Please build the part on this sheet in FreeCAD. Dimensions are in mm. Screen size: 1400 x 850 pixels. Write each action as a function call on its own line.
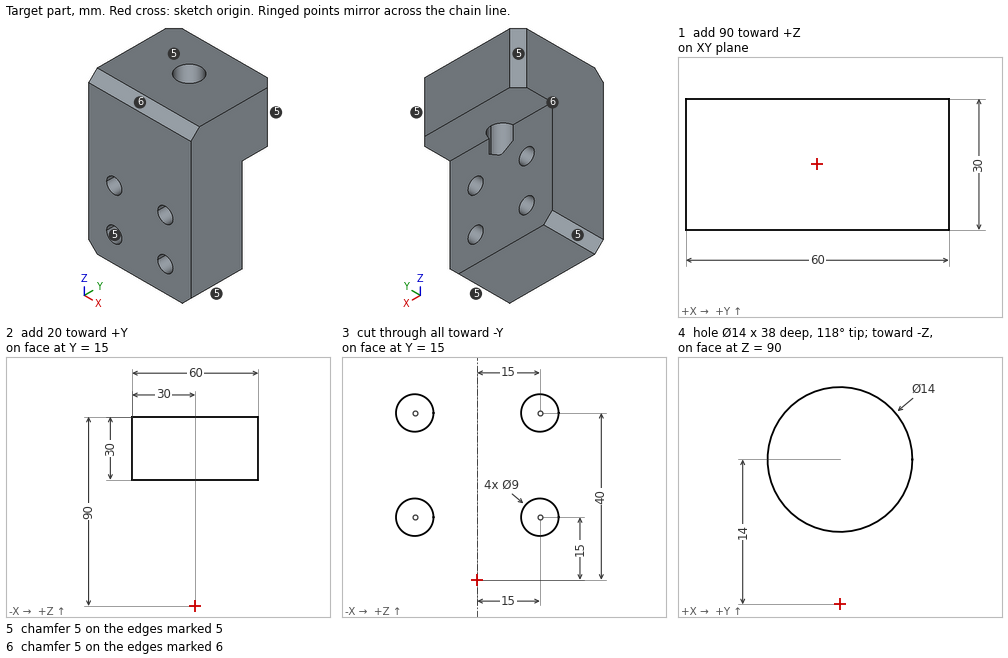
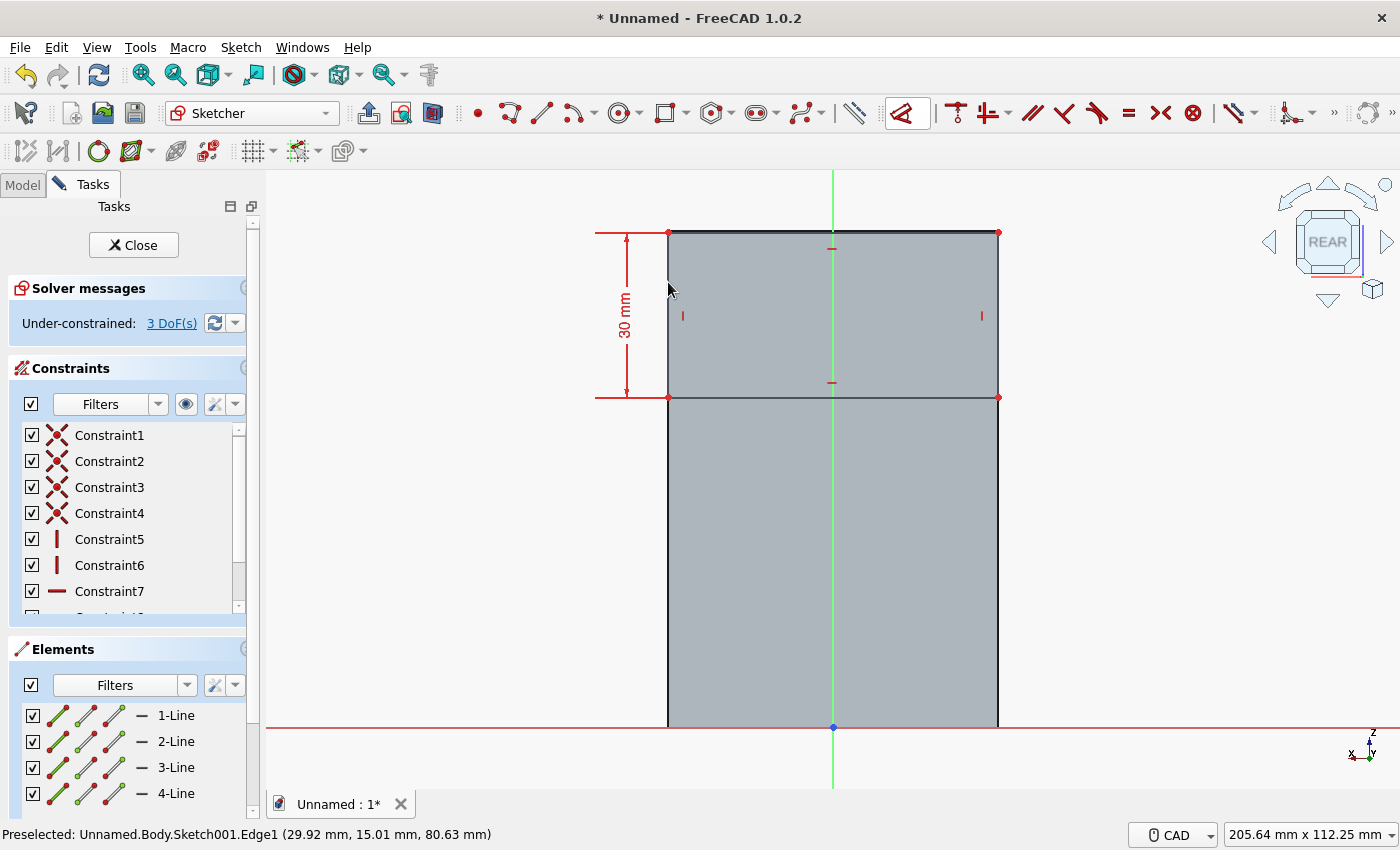
click(767, 398)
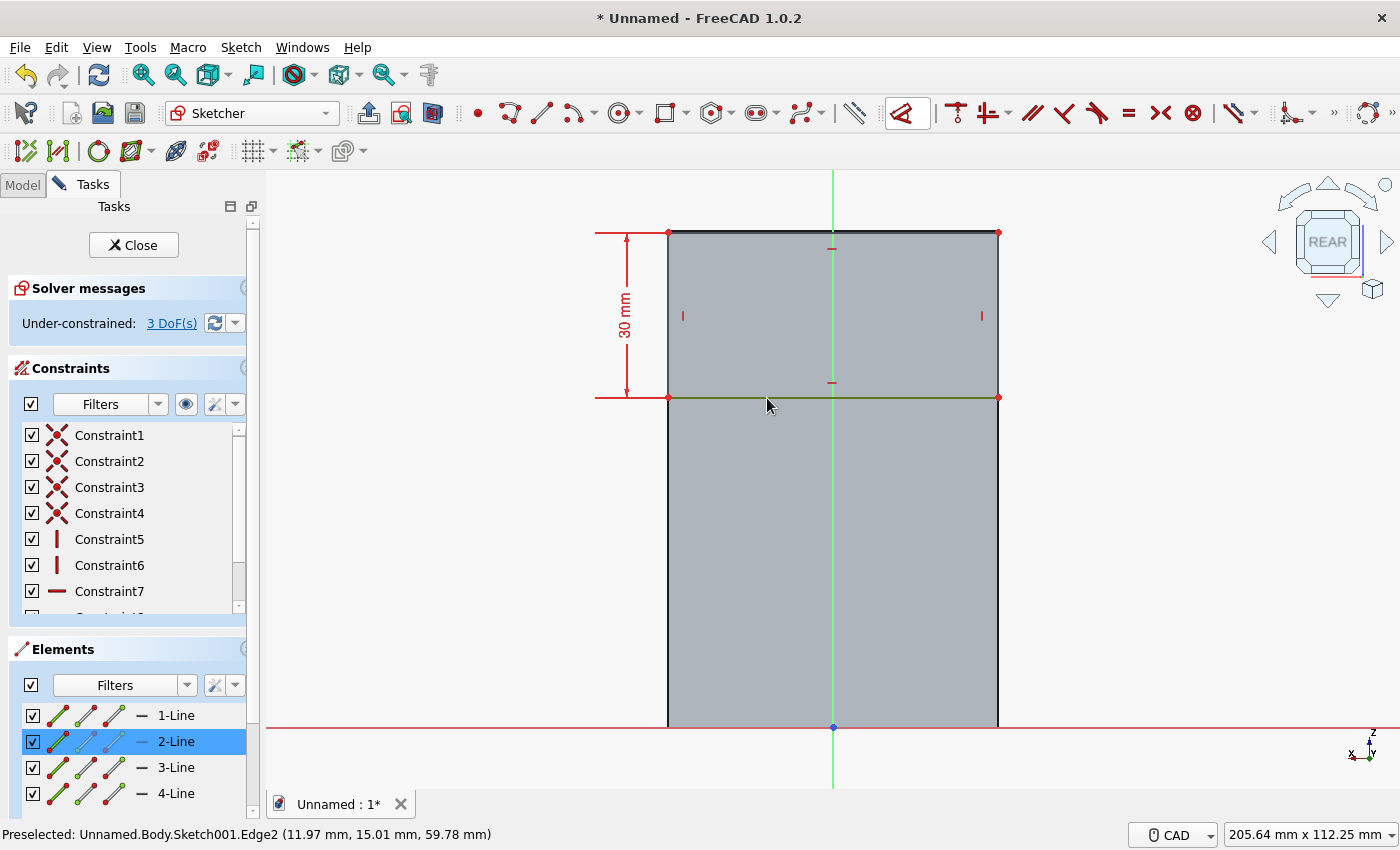
key(l)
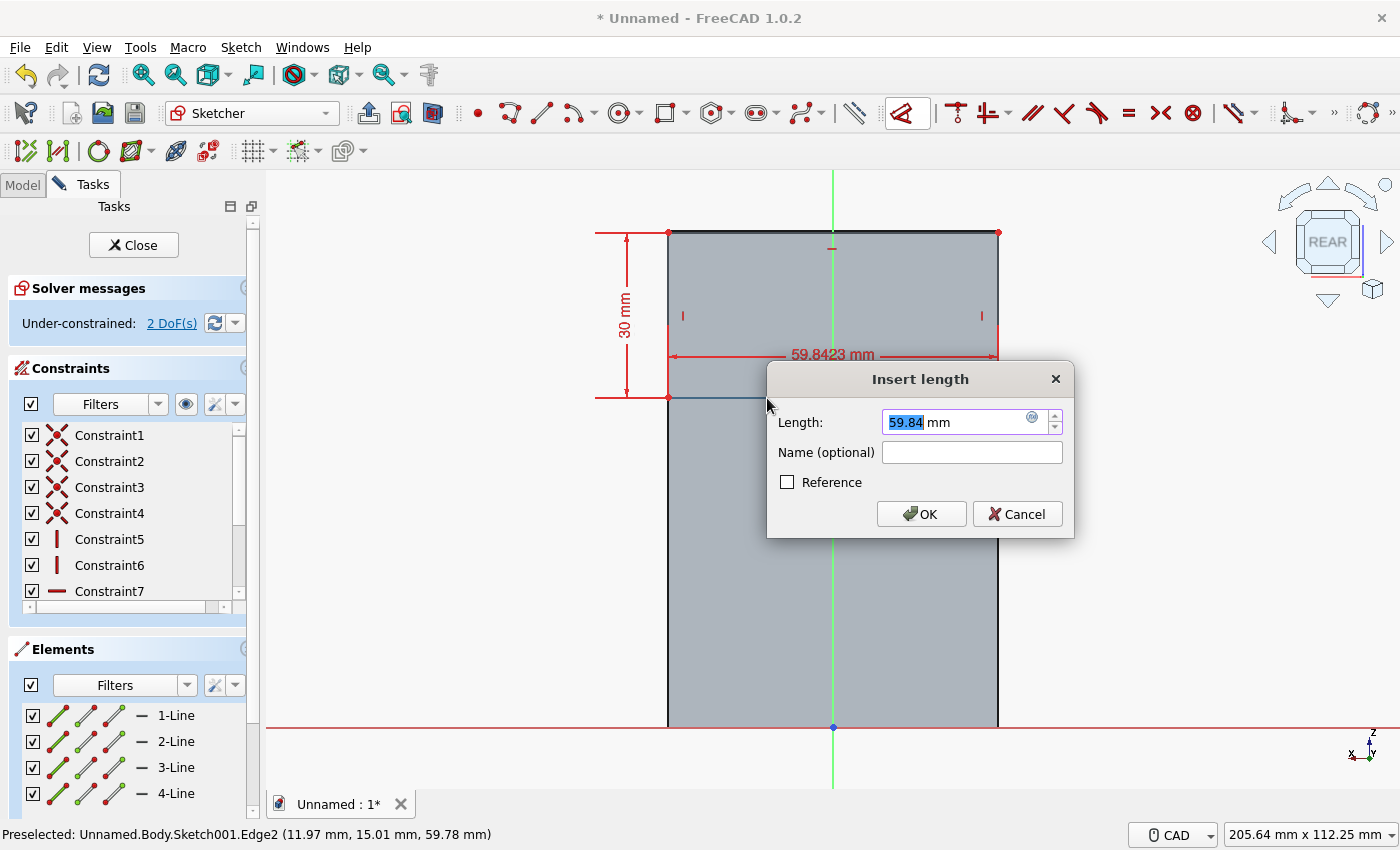
text(60)
key(Return)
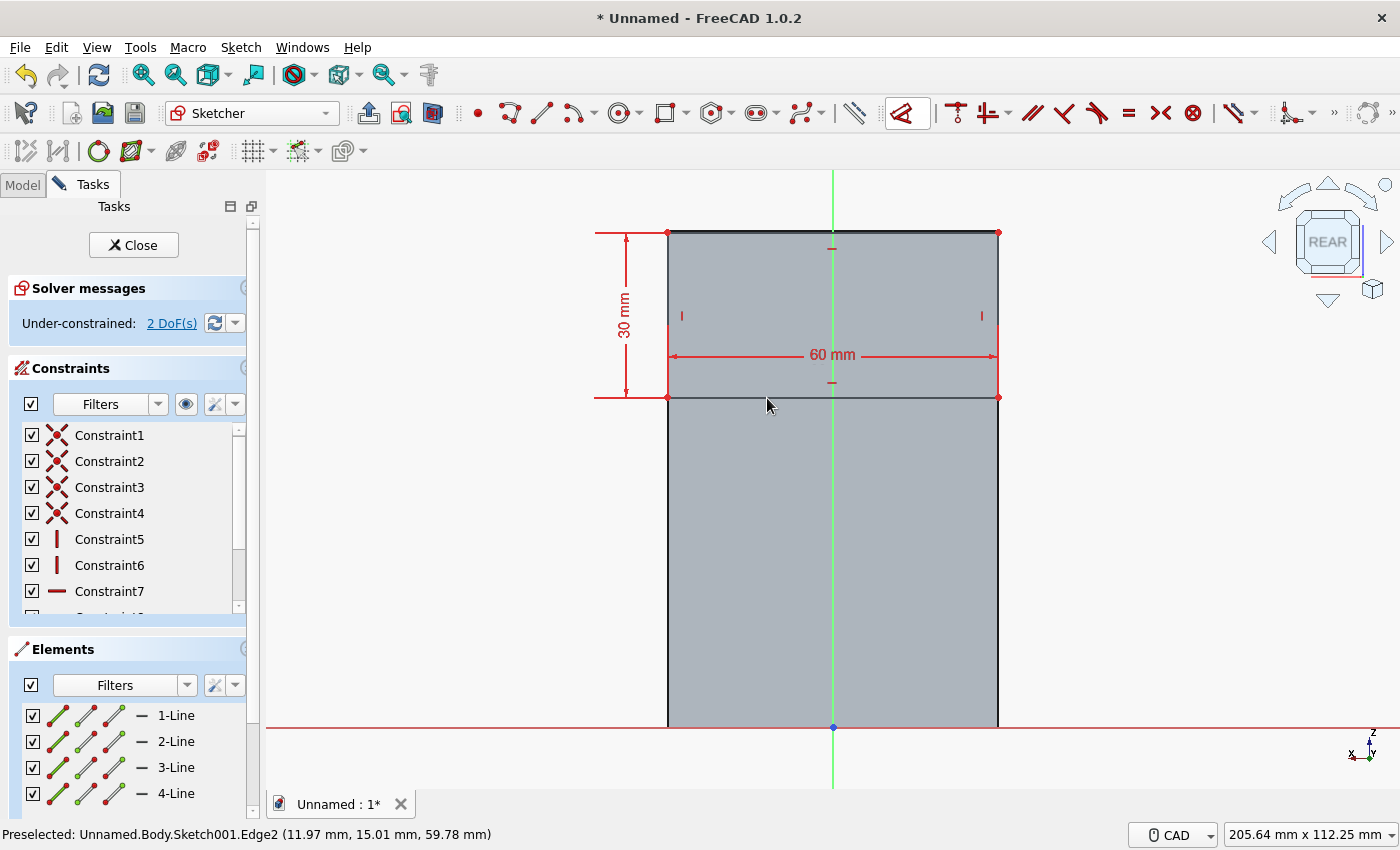
click(668, 233)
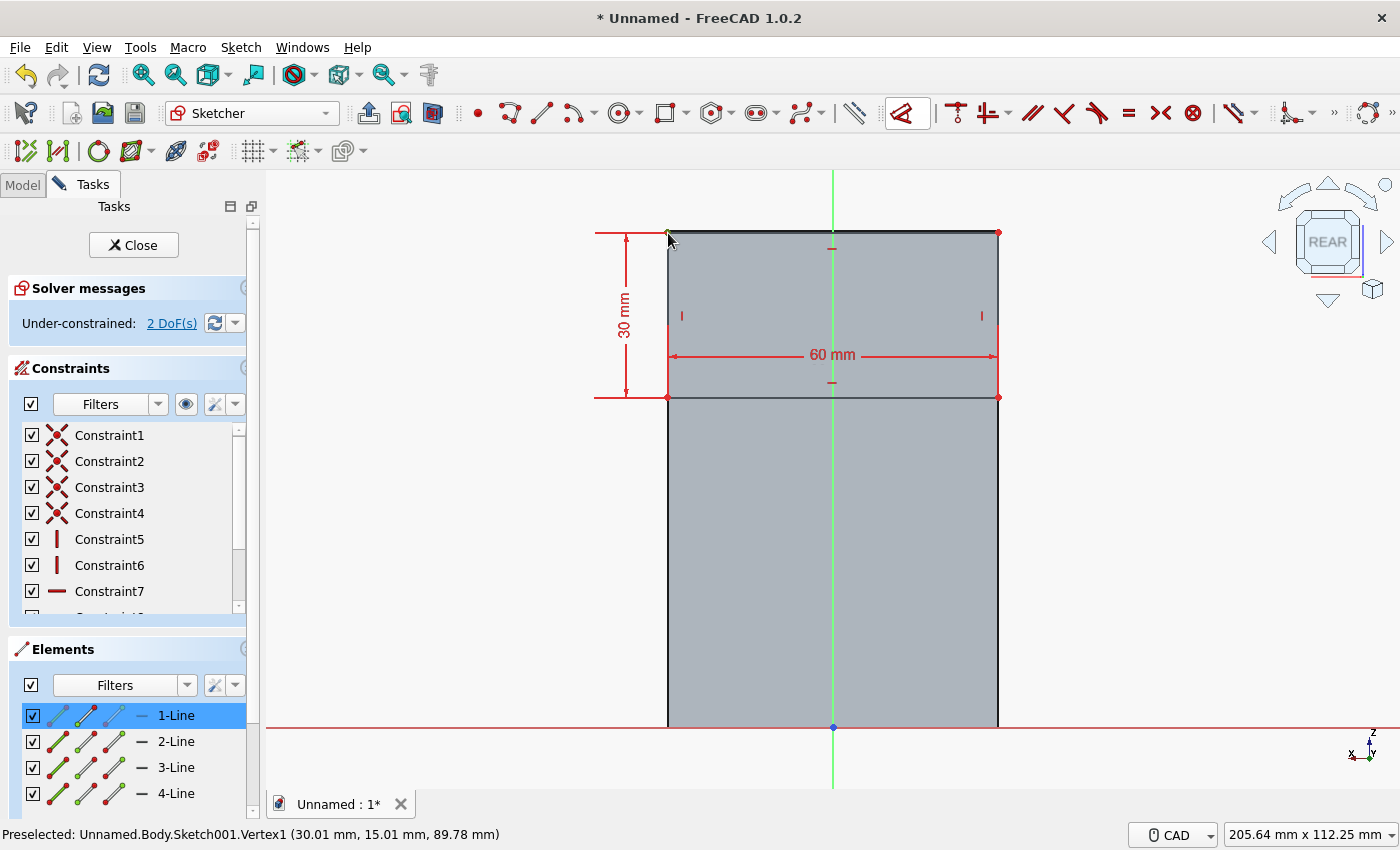
key(l)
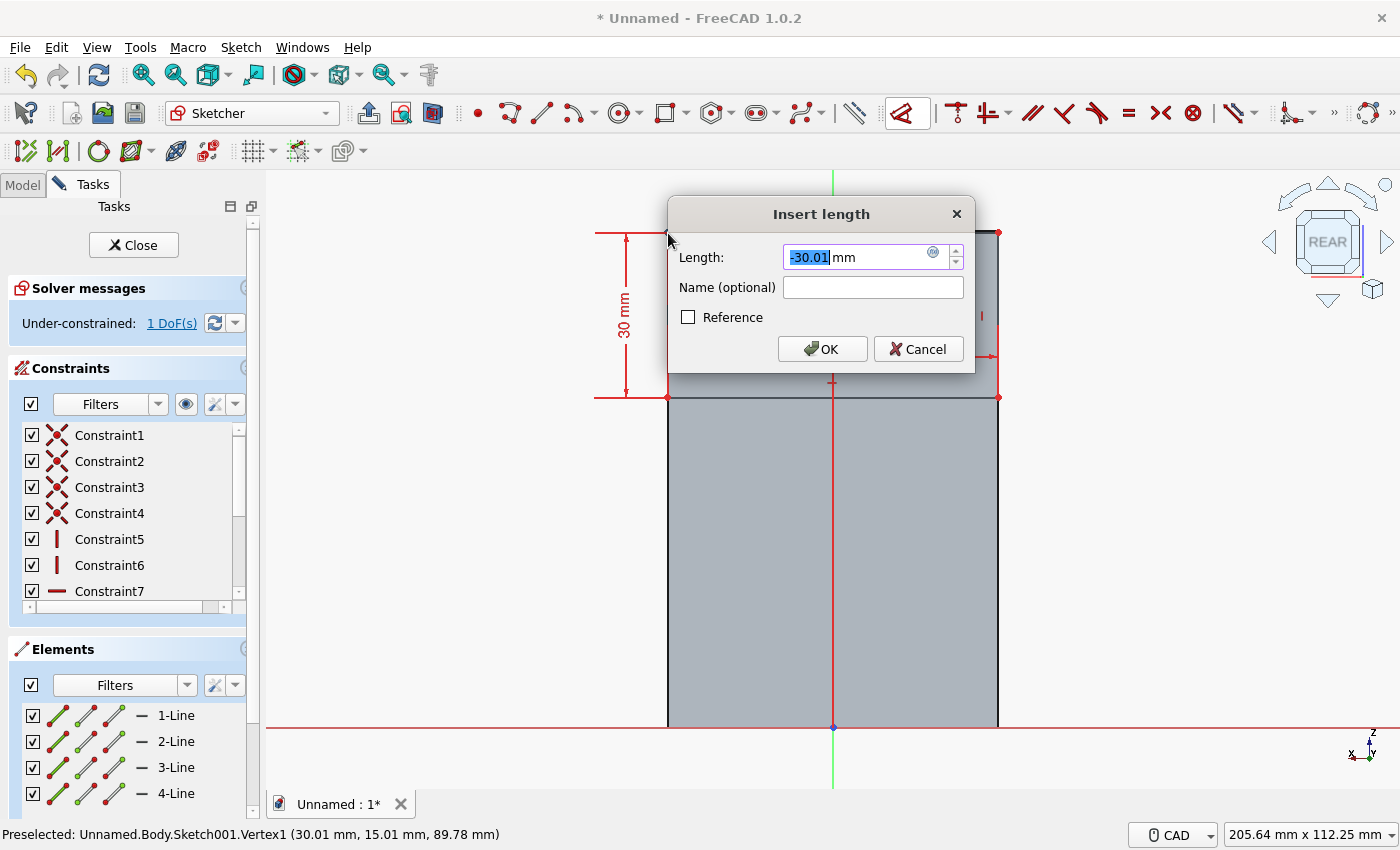
text(-30)
key(Return)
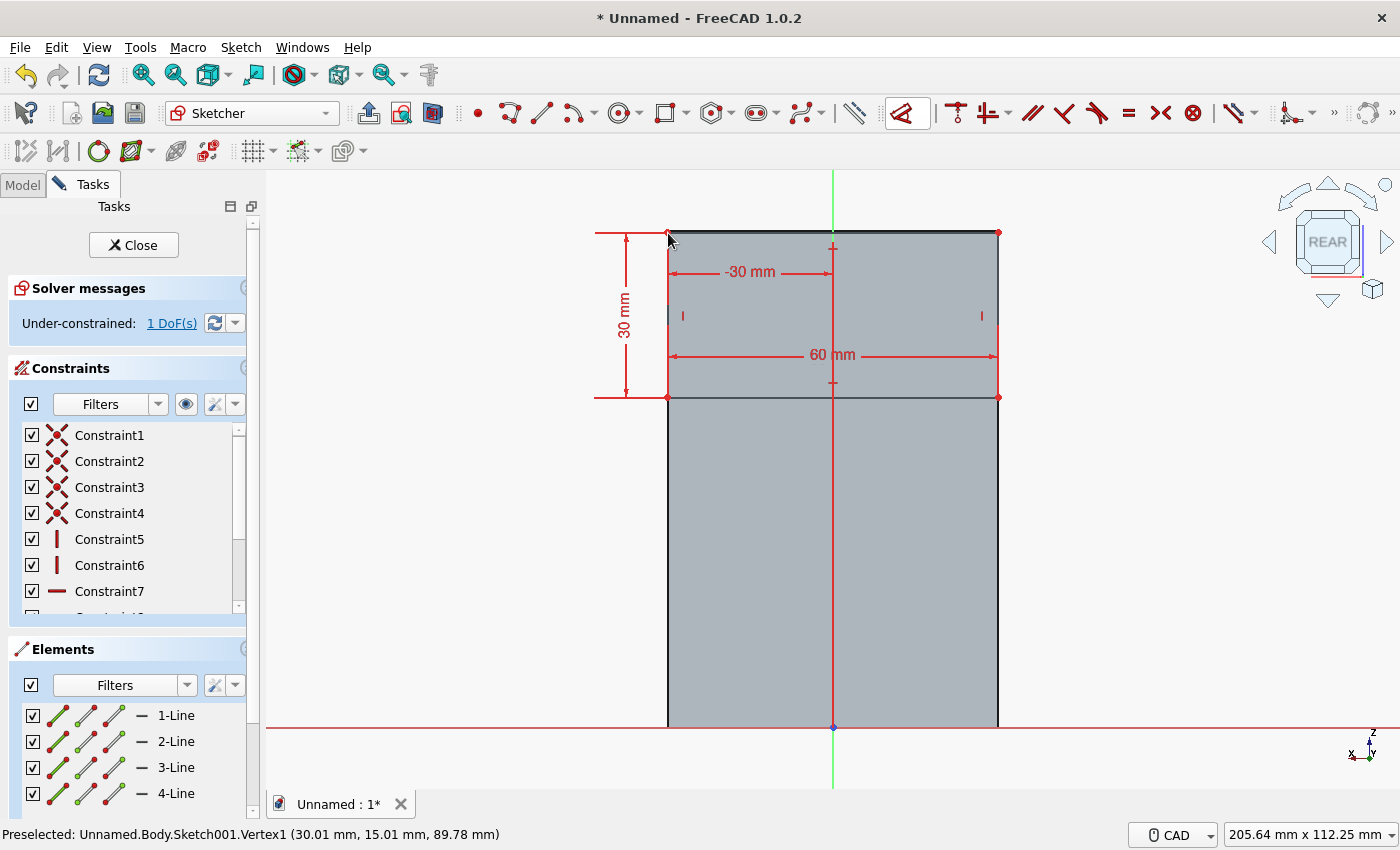
click(668, 233)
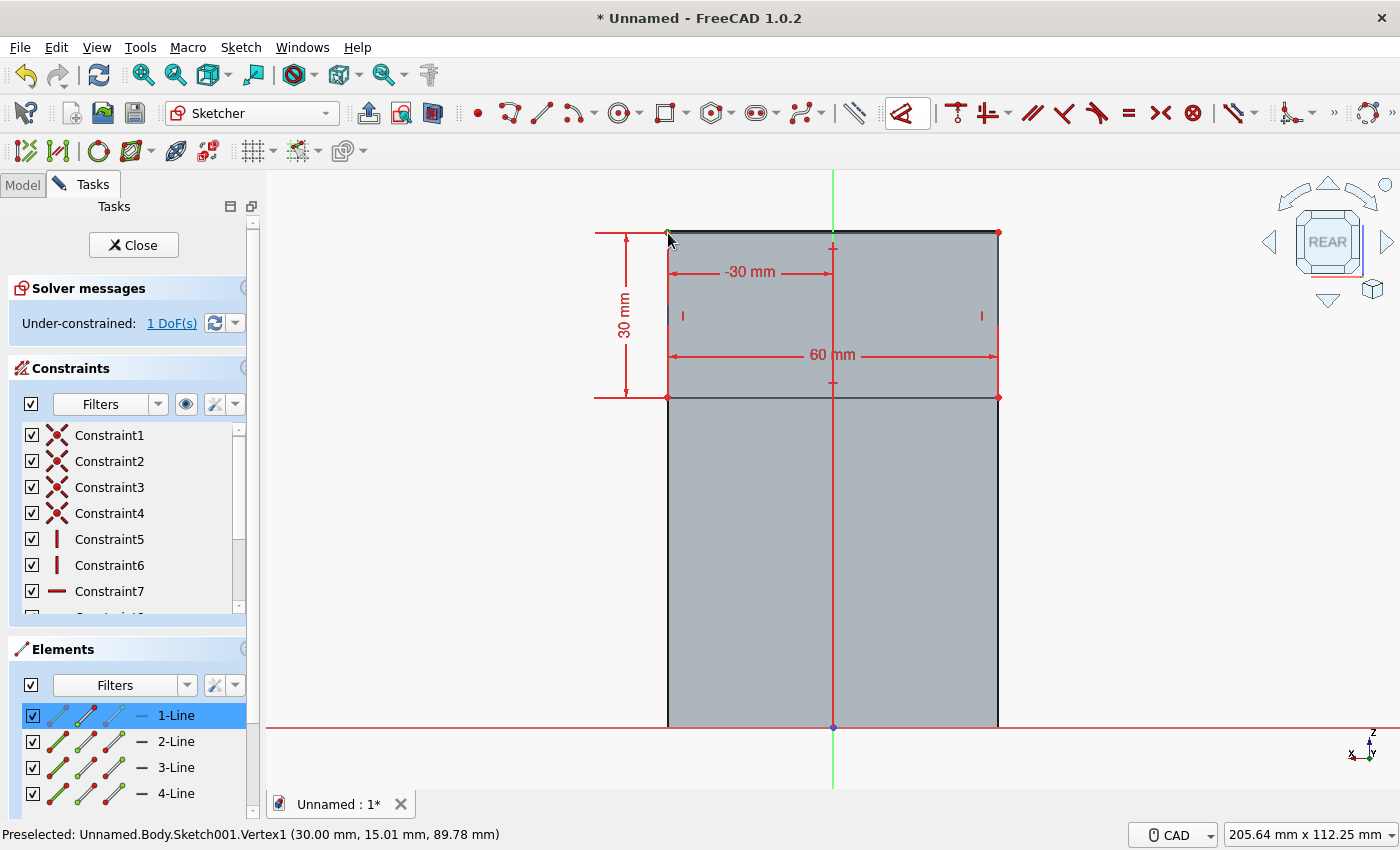
click(924, 114)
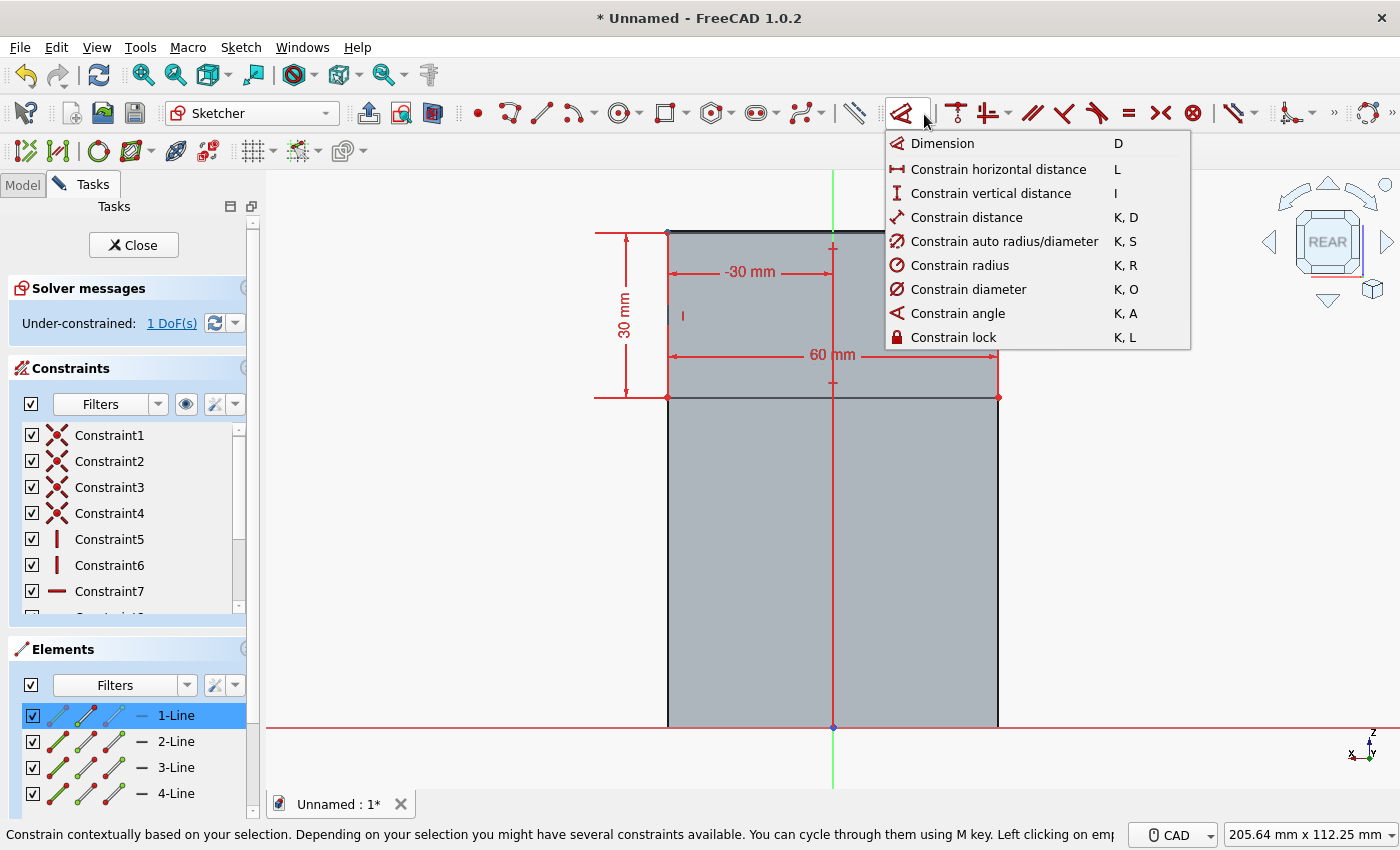
click(1038, 193)